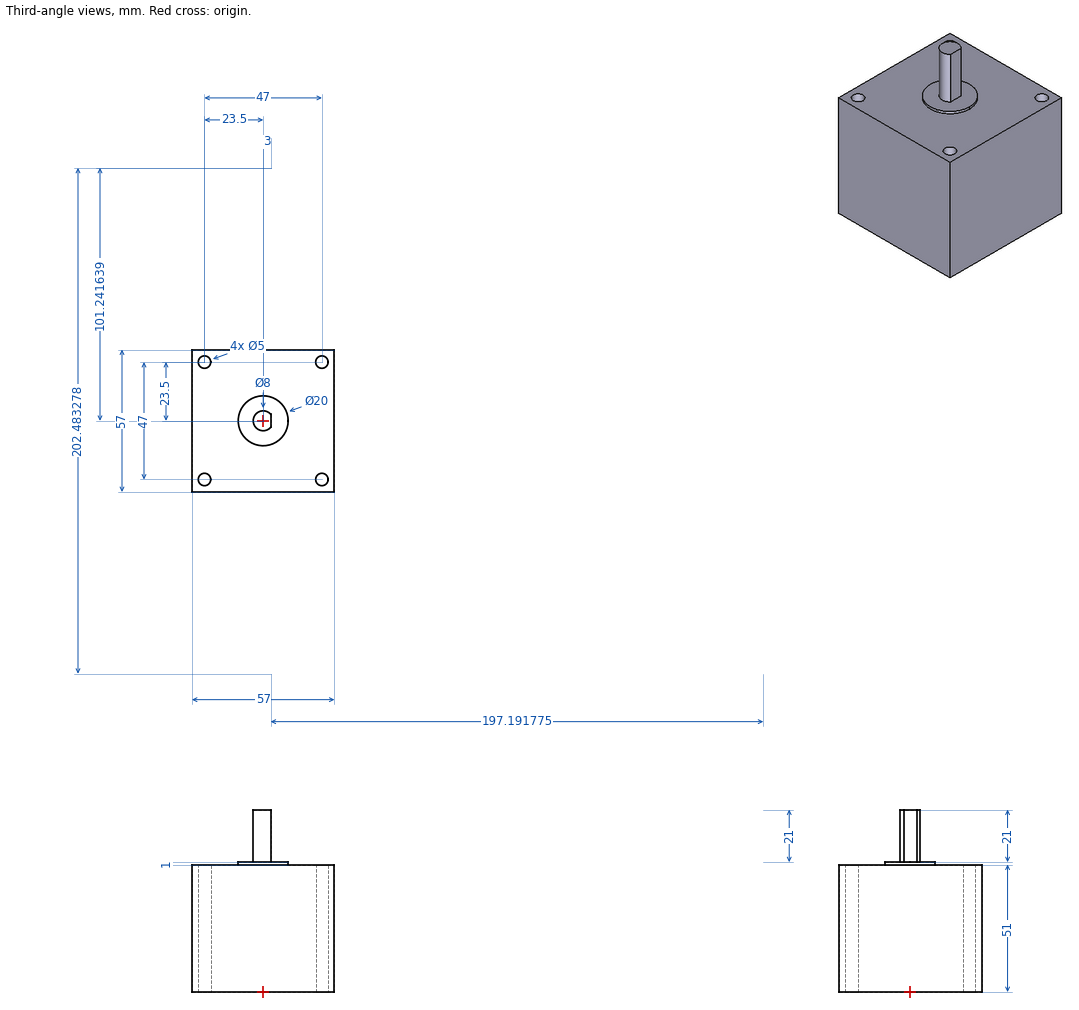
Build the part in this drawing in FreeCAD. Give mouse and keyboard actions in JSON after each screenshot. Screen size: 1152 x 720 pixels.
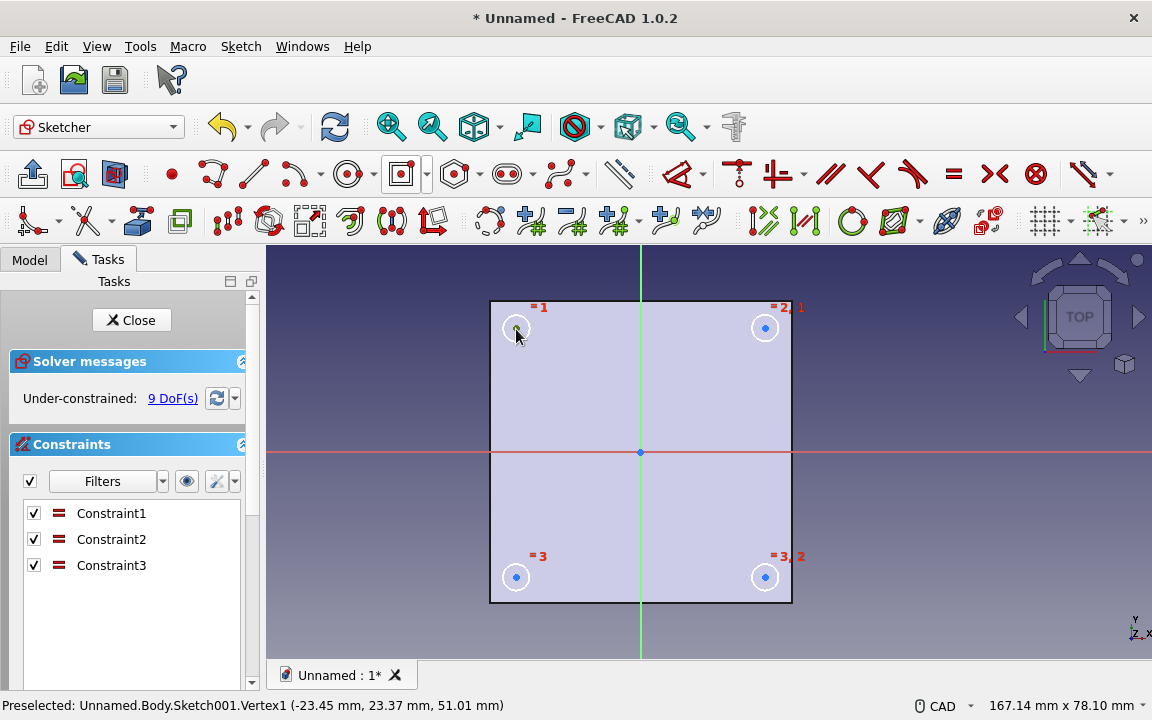
{"action": "left_click", "coordinate": [765, 328]}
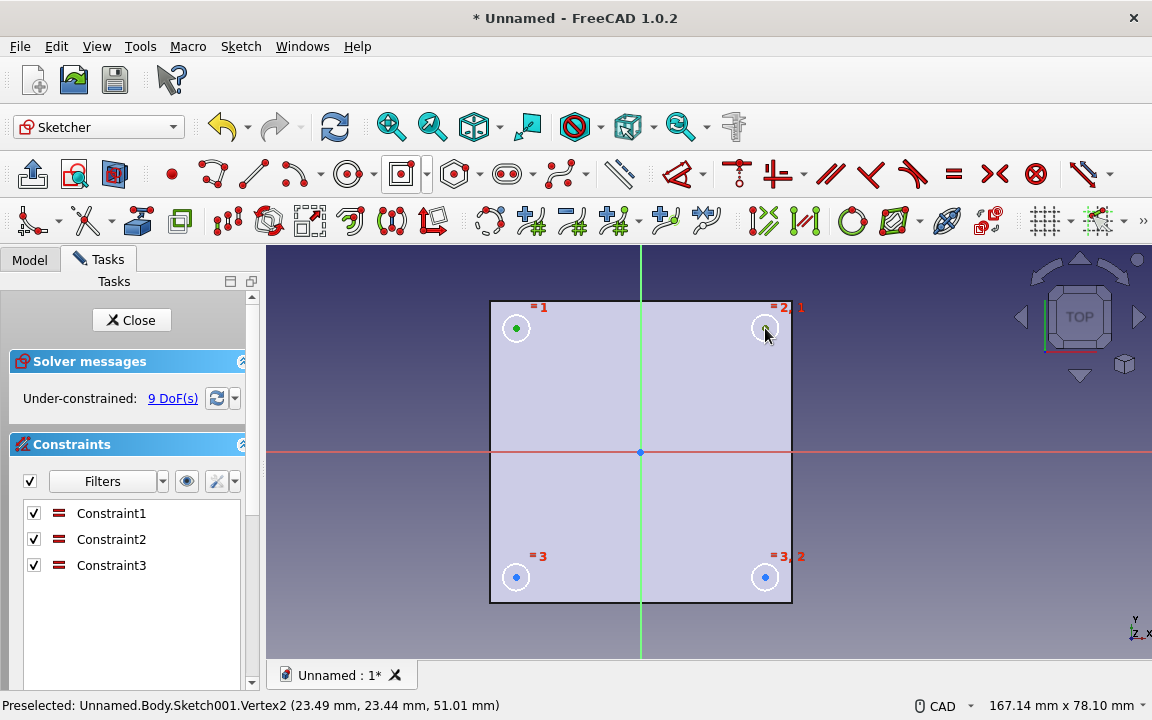
{"action": "left_click", "coordinate": [804, 174]}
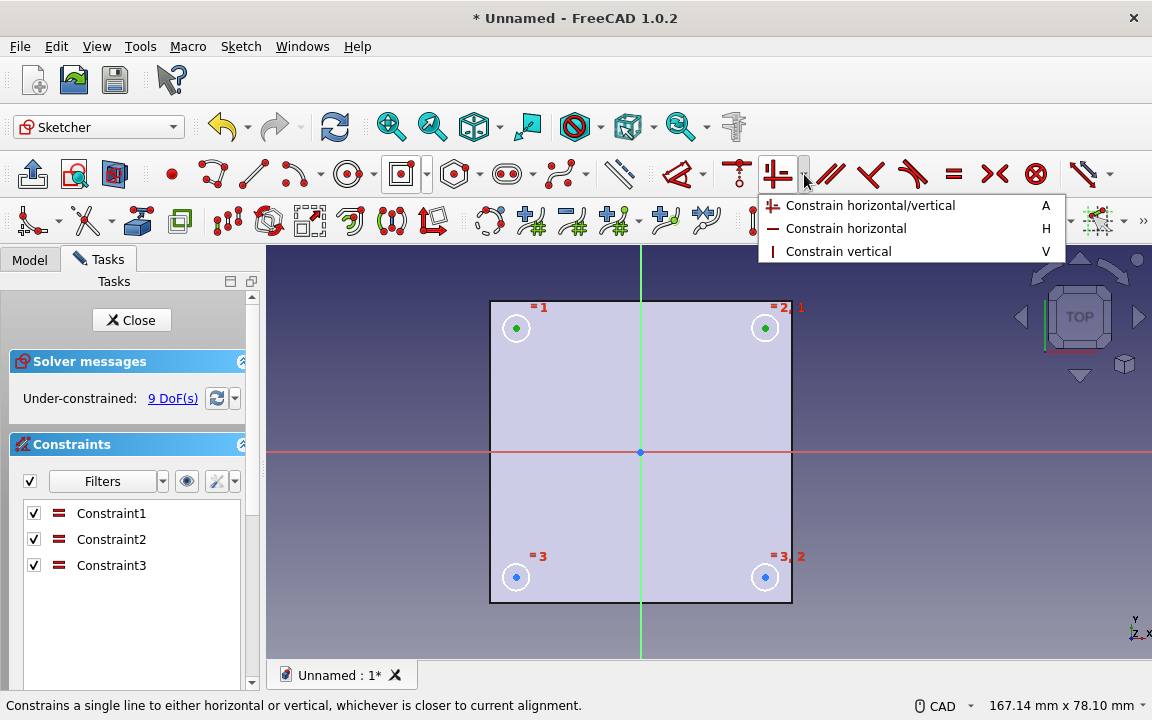
{"action": "left_click", "coordinate": [912, 228]}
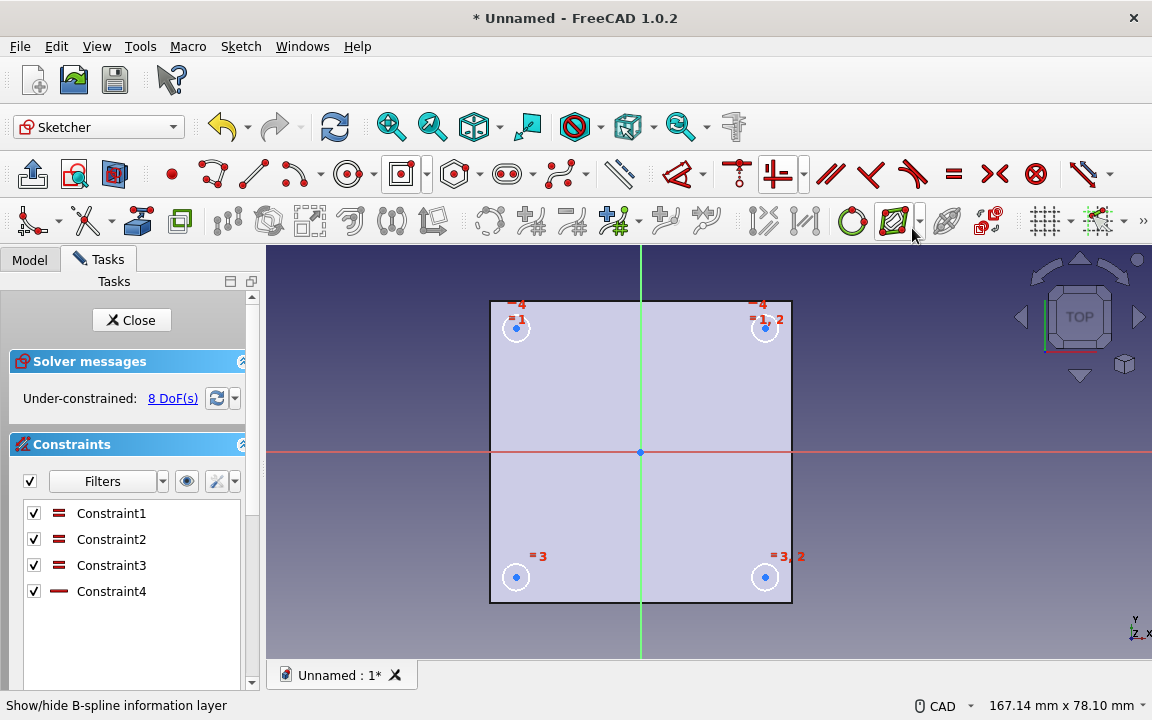
{"action": "left_click", "coordinate": [765, 329]}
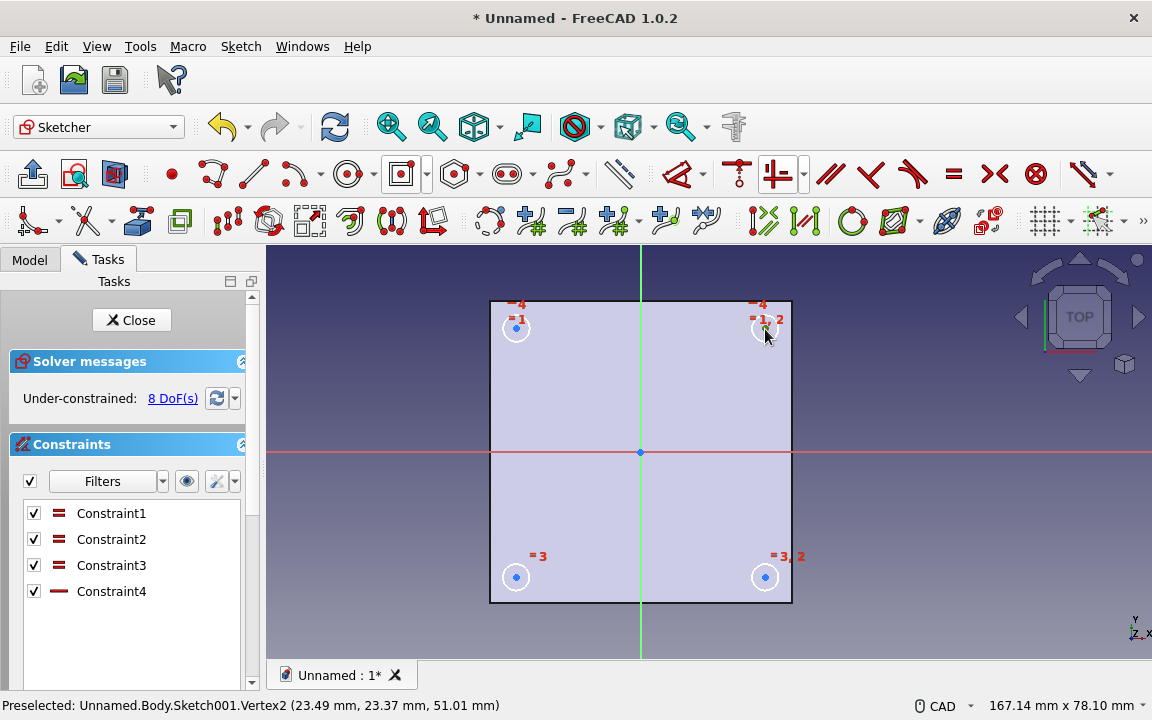
{"action": "left_click", "coordinate": [765, 577]}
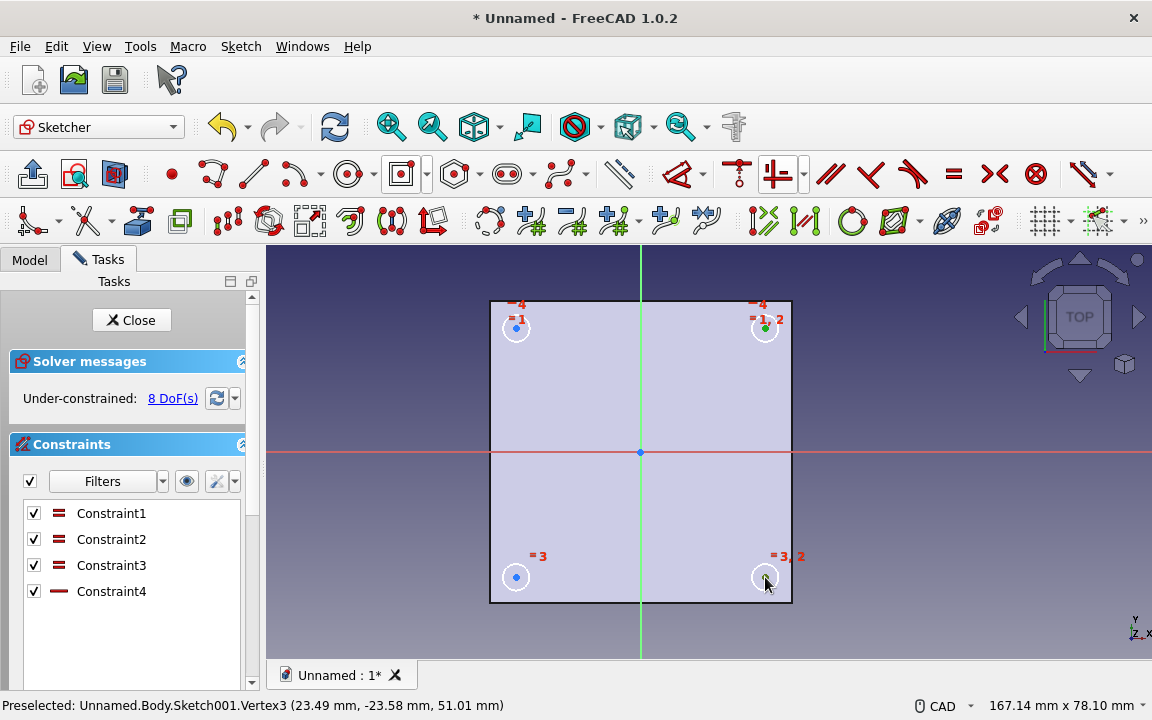
{"action": "key", "text": "v"}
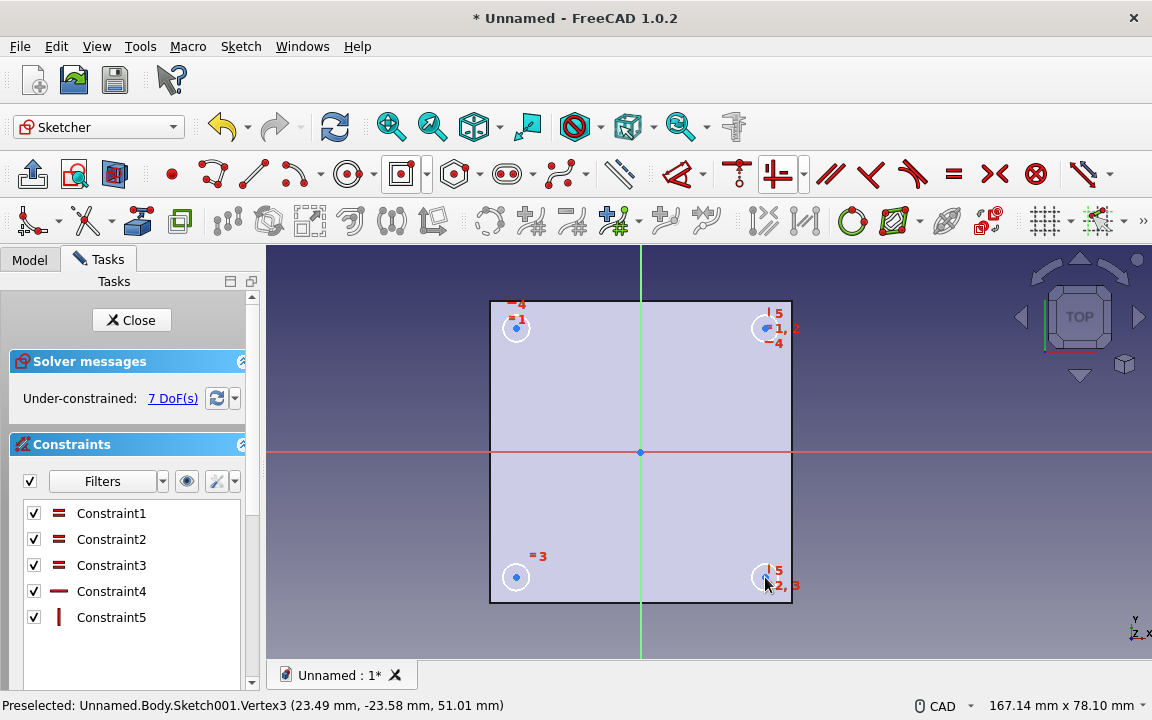
{"action": "left_click", "coordinate": [516, 329]}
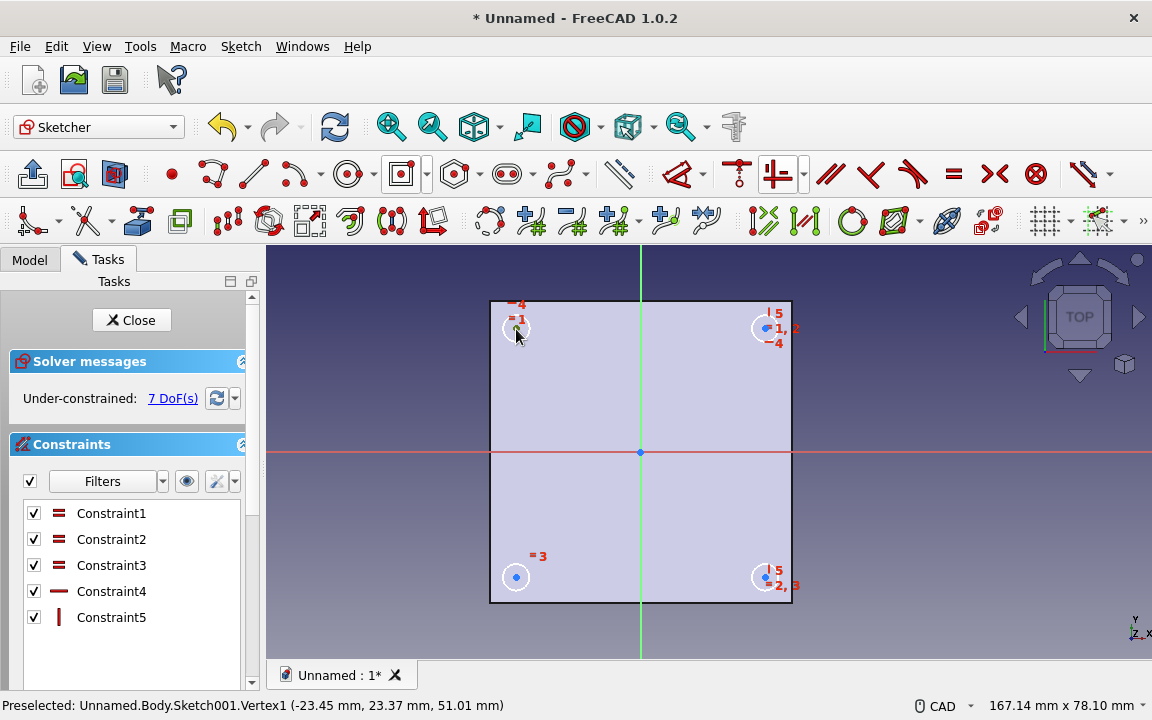
{"action": "left_click", "coordinate": [516, 577]}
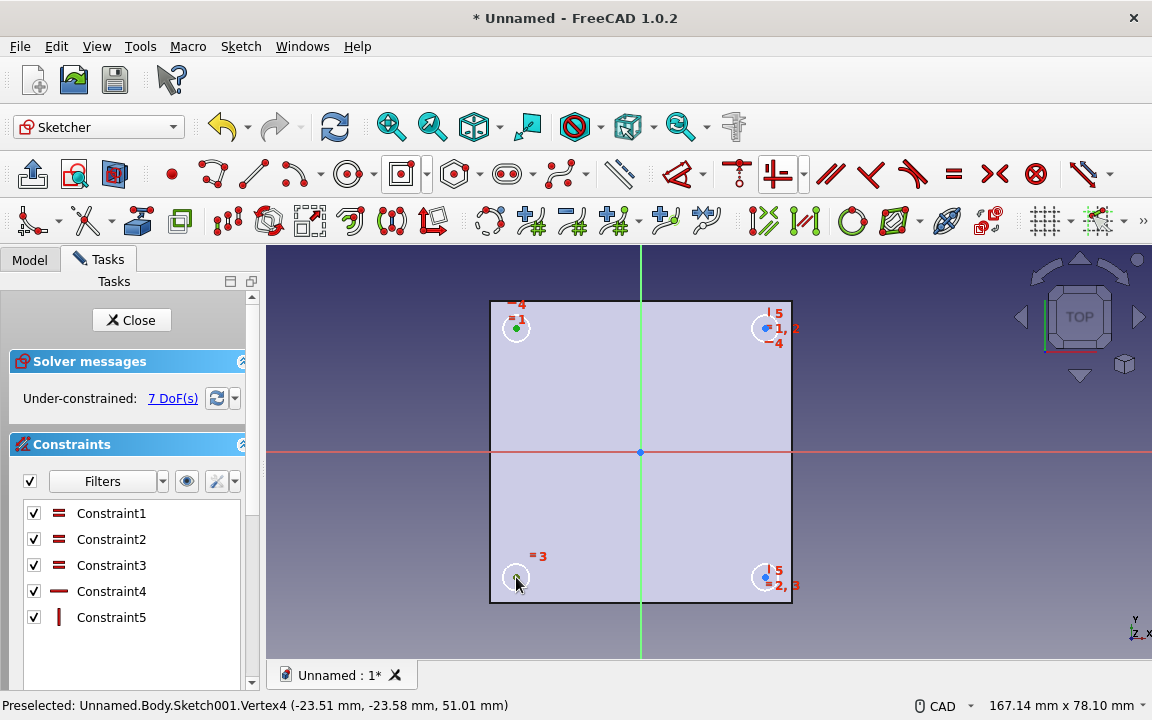
{"action": "left_click", "coordinate": [804, 174]}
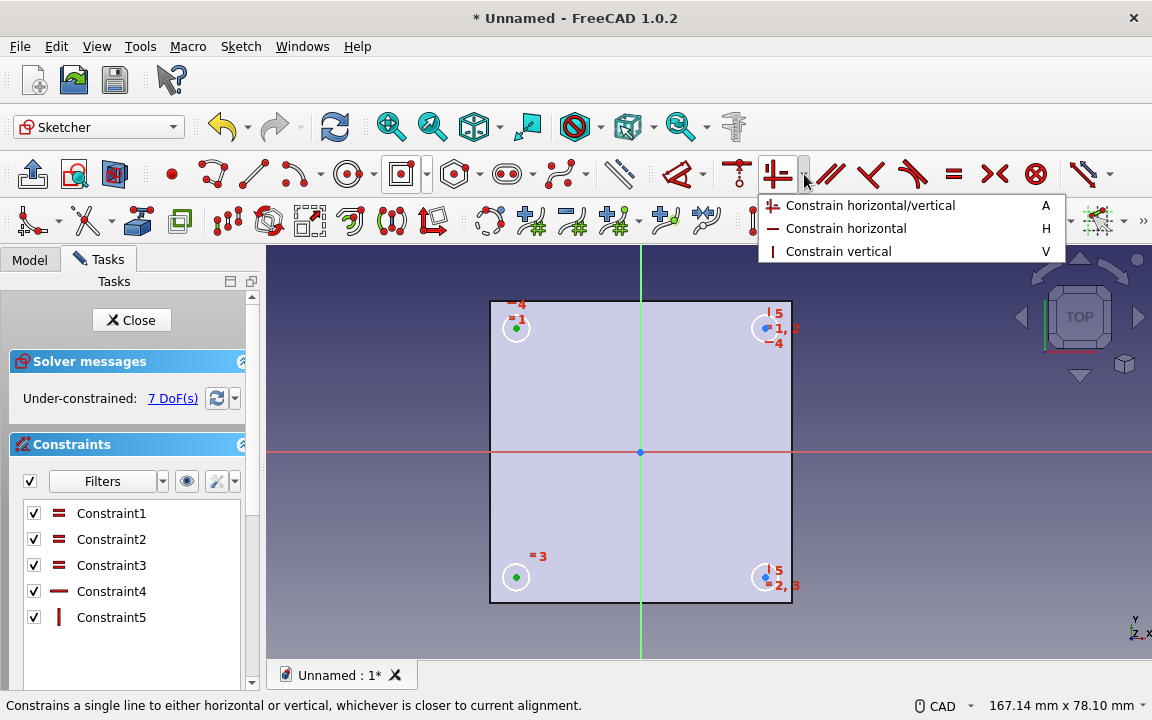
{"action": "left_click", "coordinate": [912, 252]}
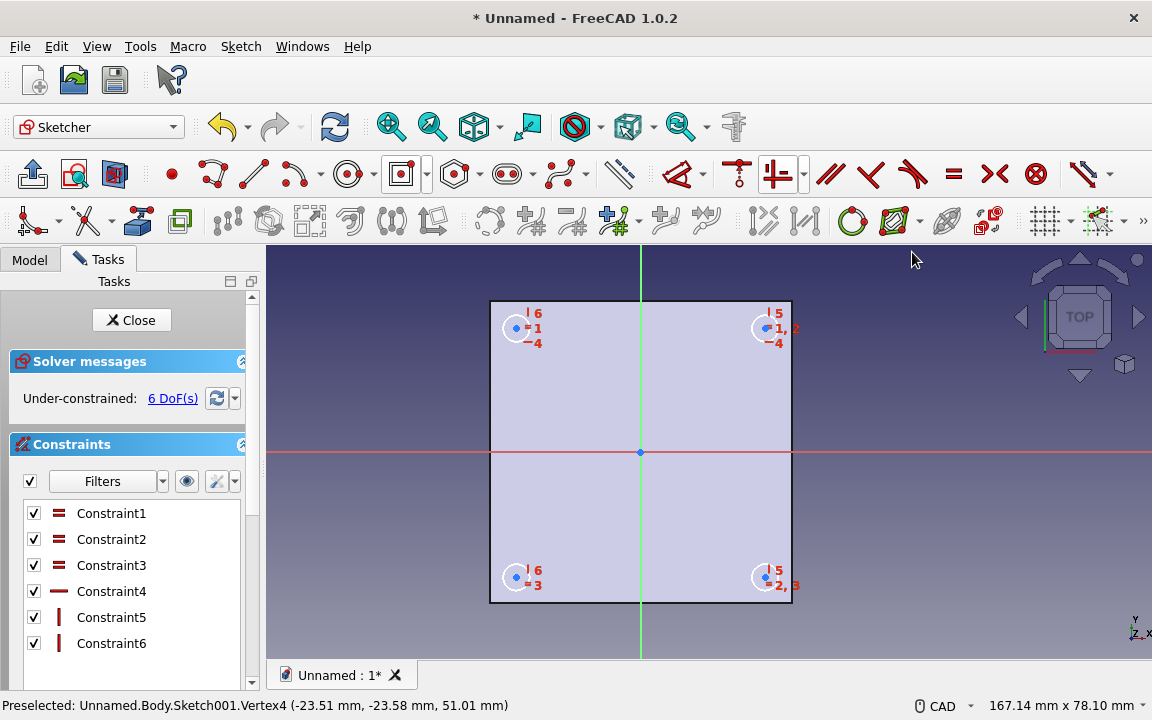
{"action": "left_click", "coordinate": [763, 579]}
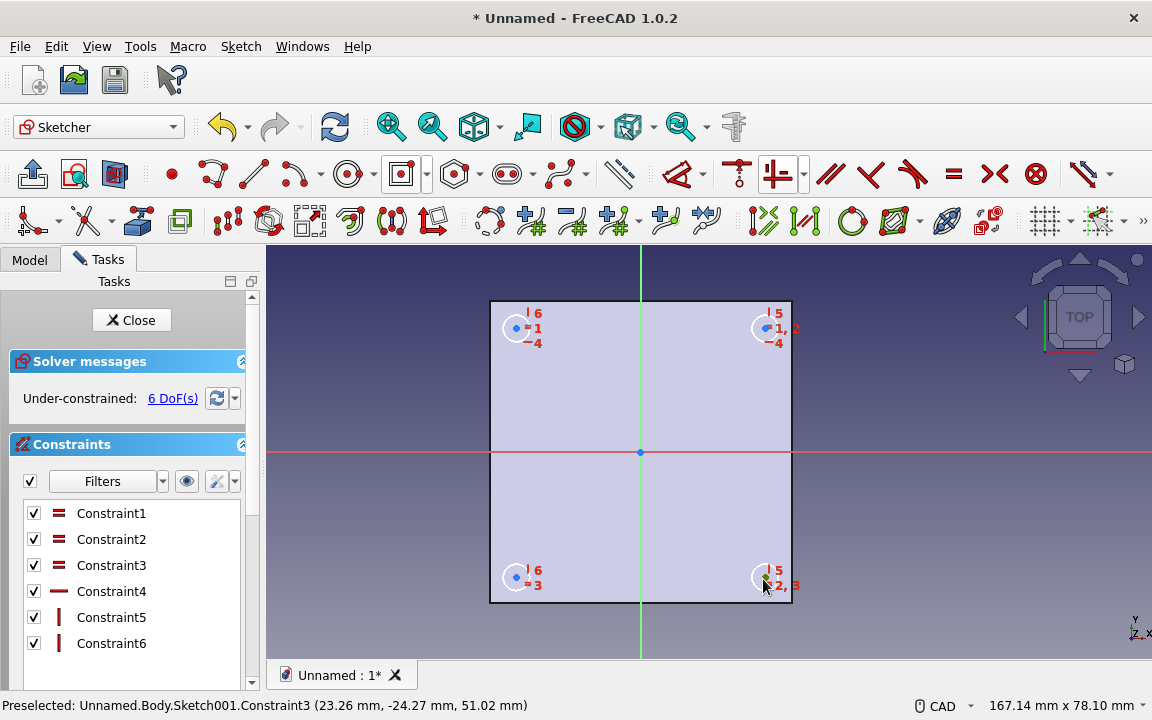
{"action": "left_click", "coordinate": [516, 577]}